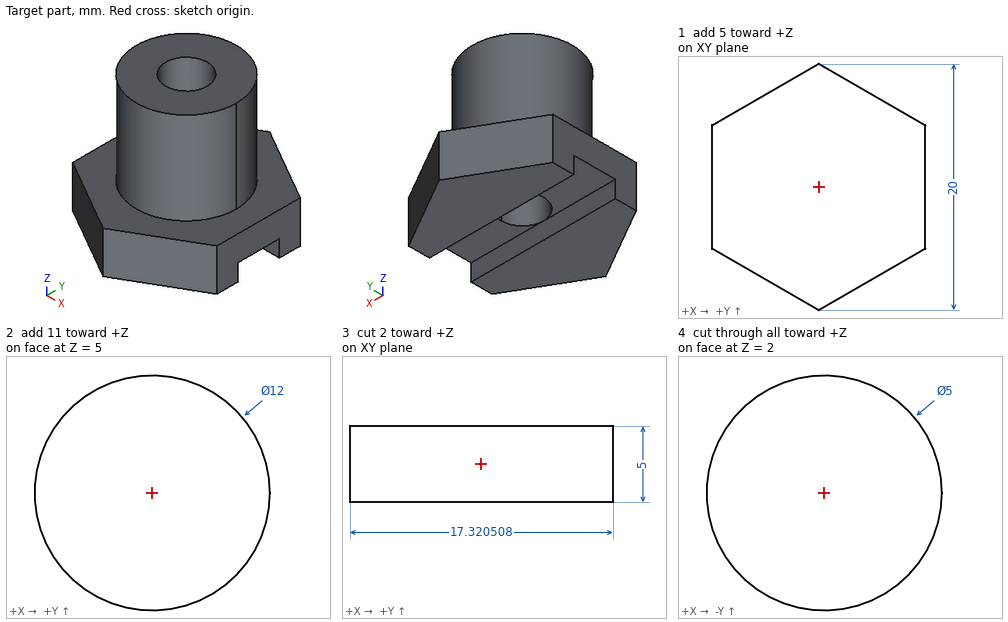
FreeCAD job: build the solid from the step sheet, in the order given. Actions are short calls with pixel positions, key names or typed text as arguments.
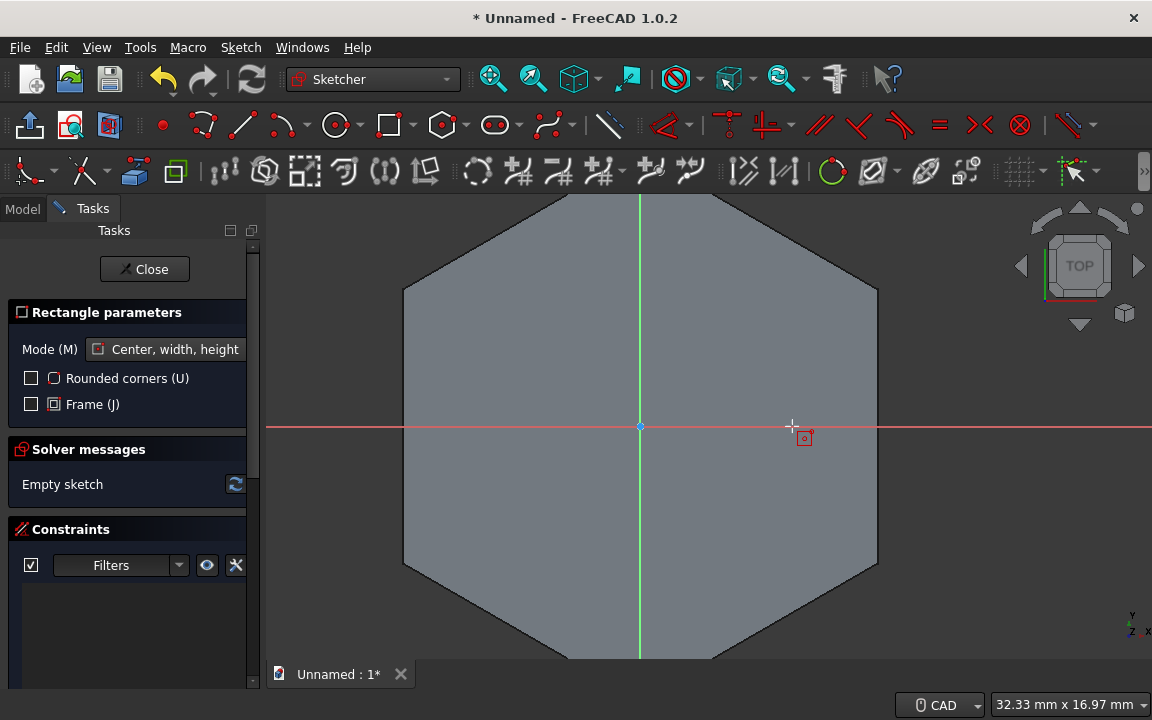
click(640, 426)
click(878, 358)
key(Escape)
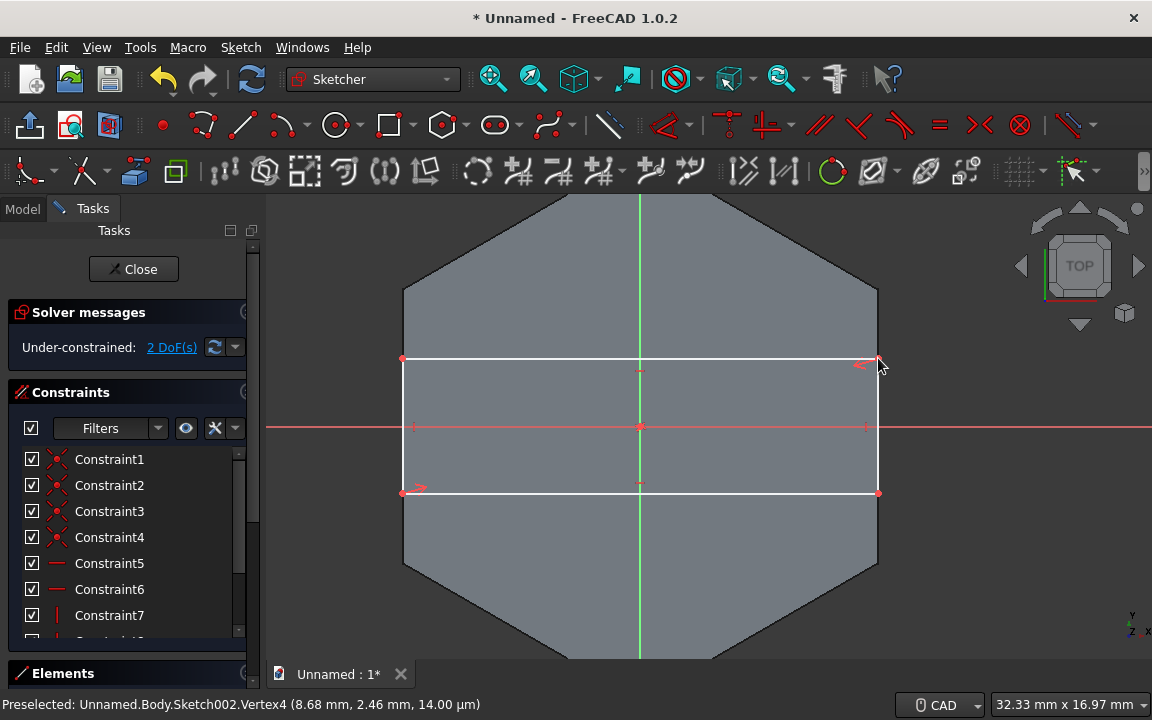
key(d)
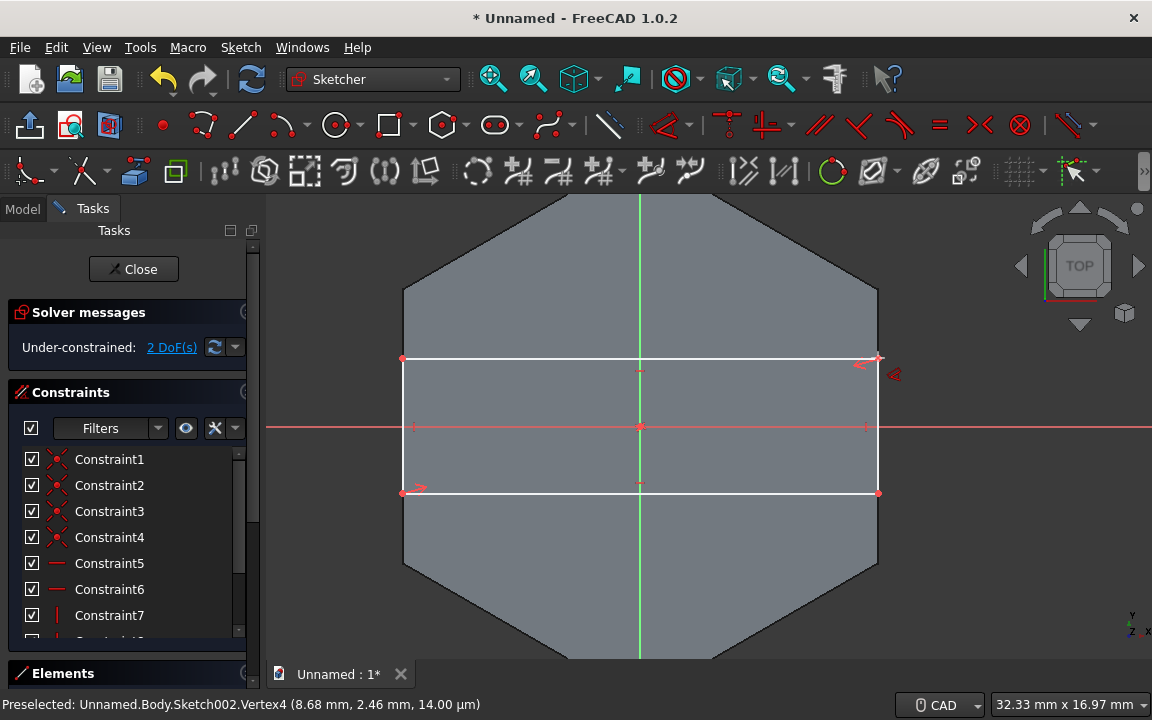
click(878, 453)
click(912, 395)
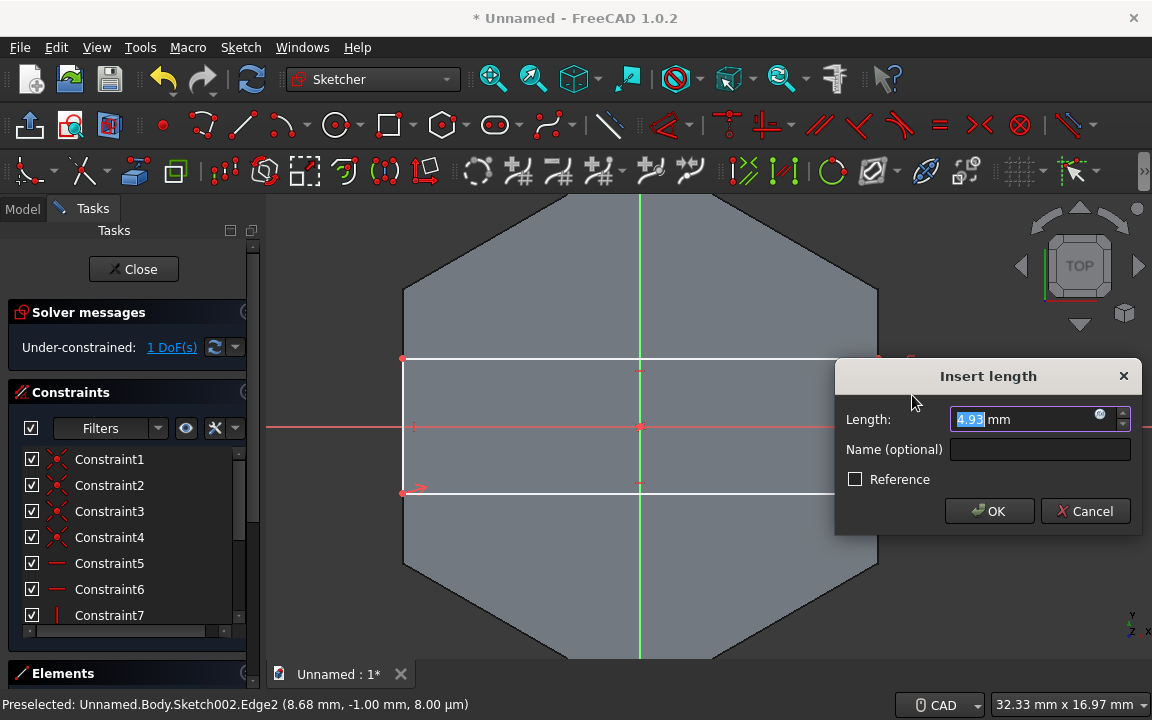
text(5)
key(Return)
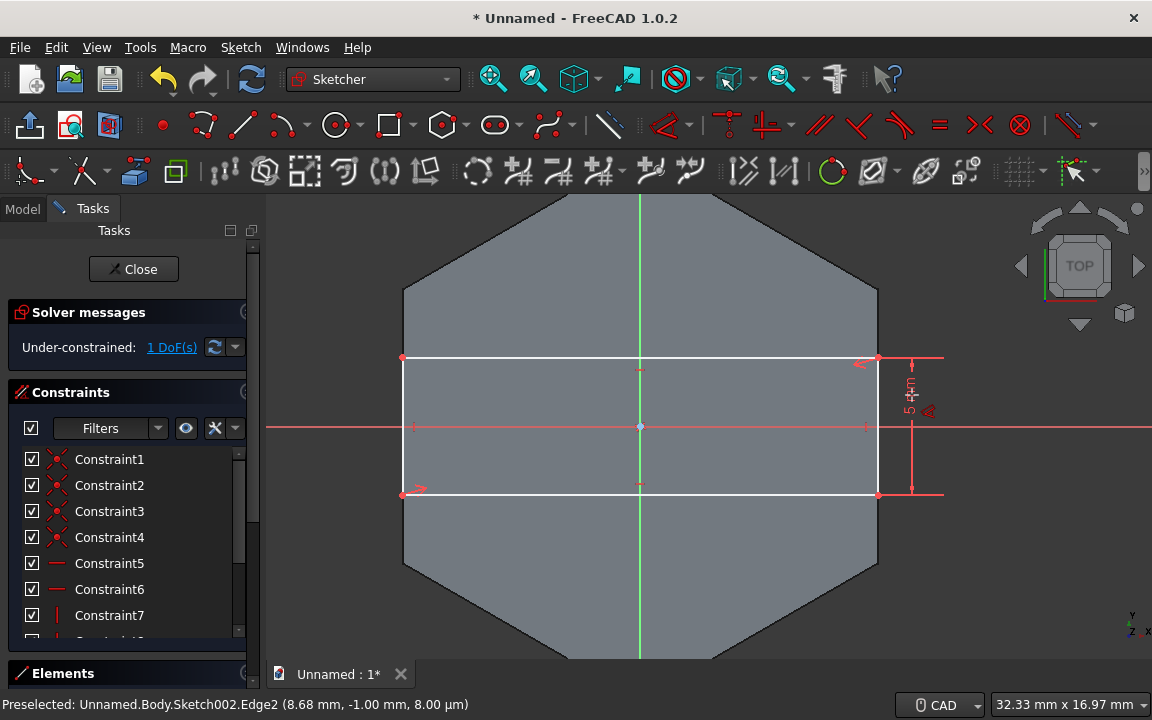
click(545, 495)
click(531, 529)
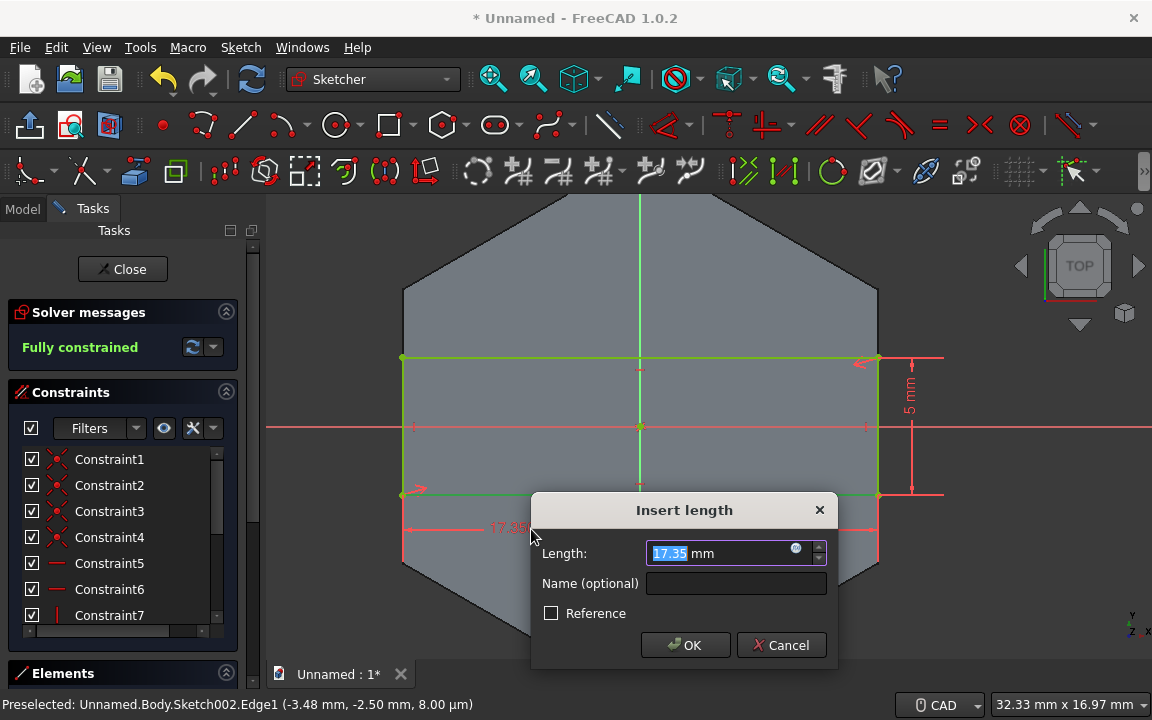
text(17.320508)
key(Return)
key(Escape)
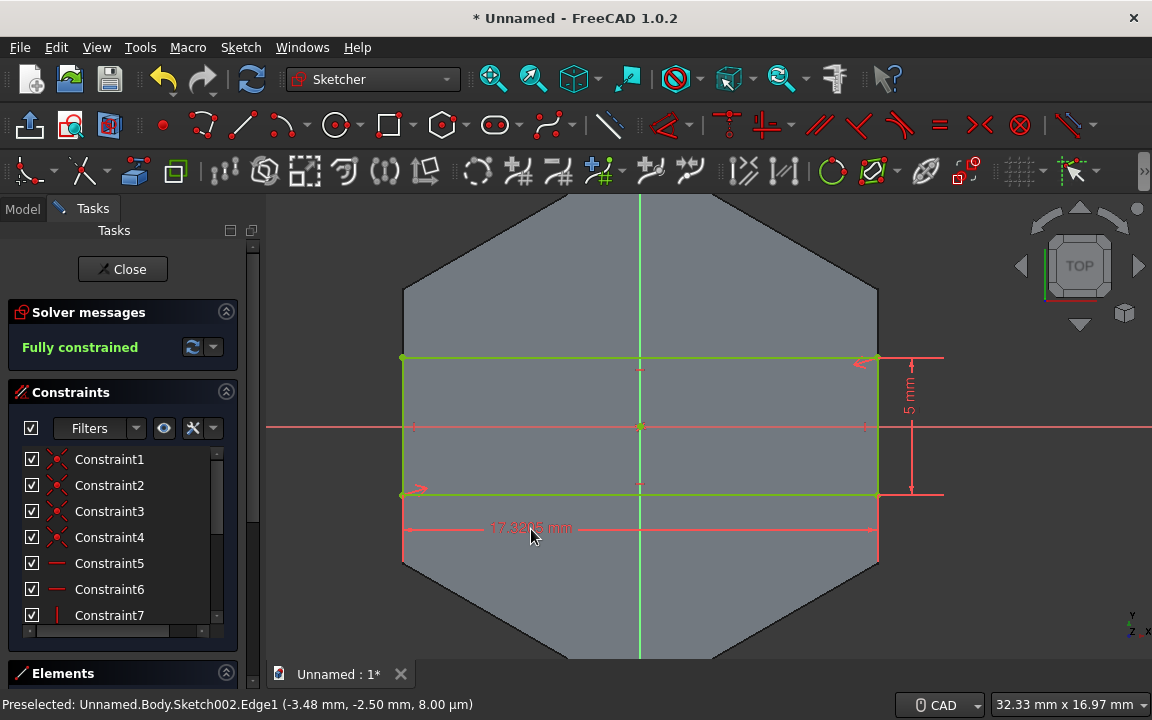
click(123, 269)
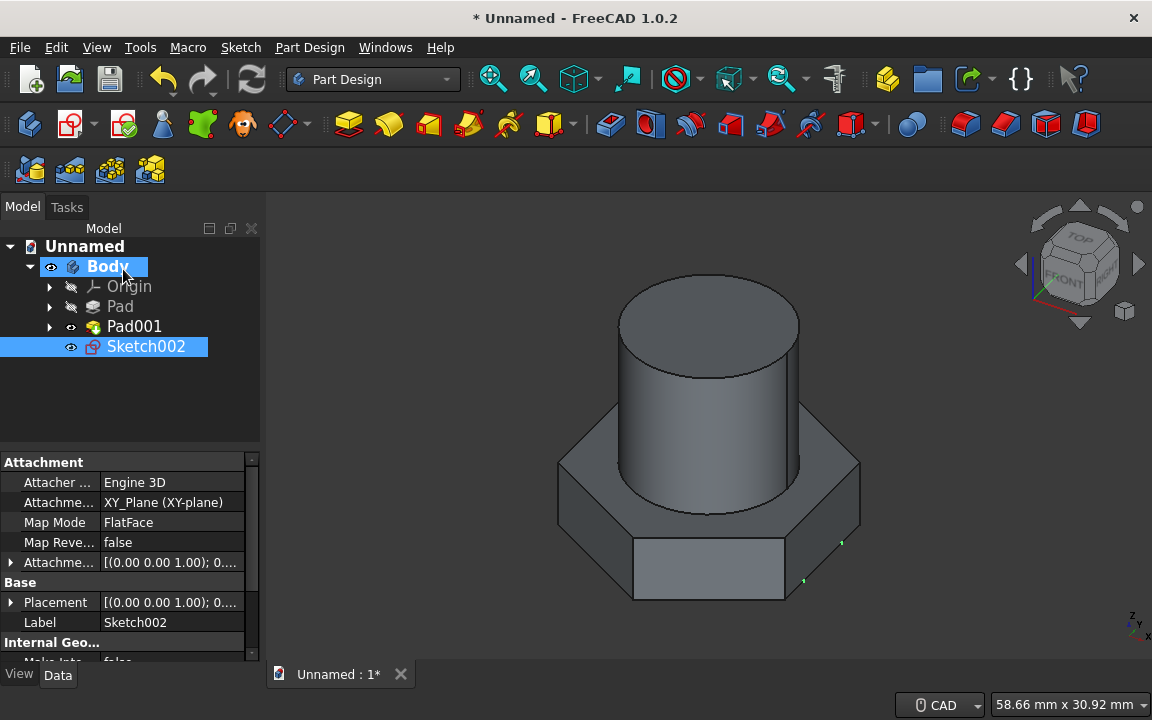
click(612, 124)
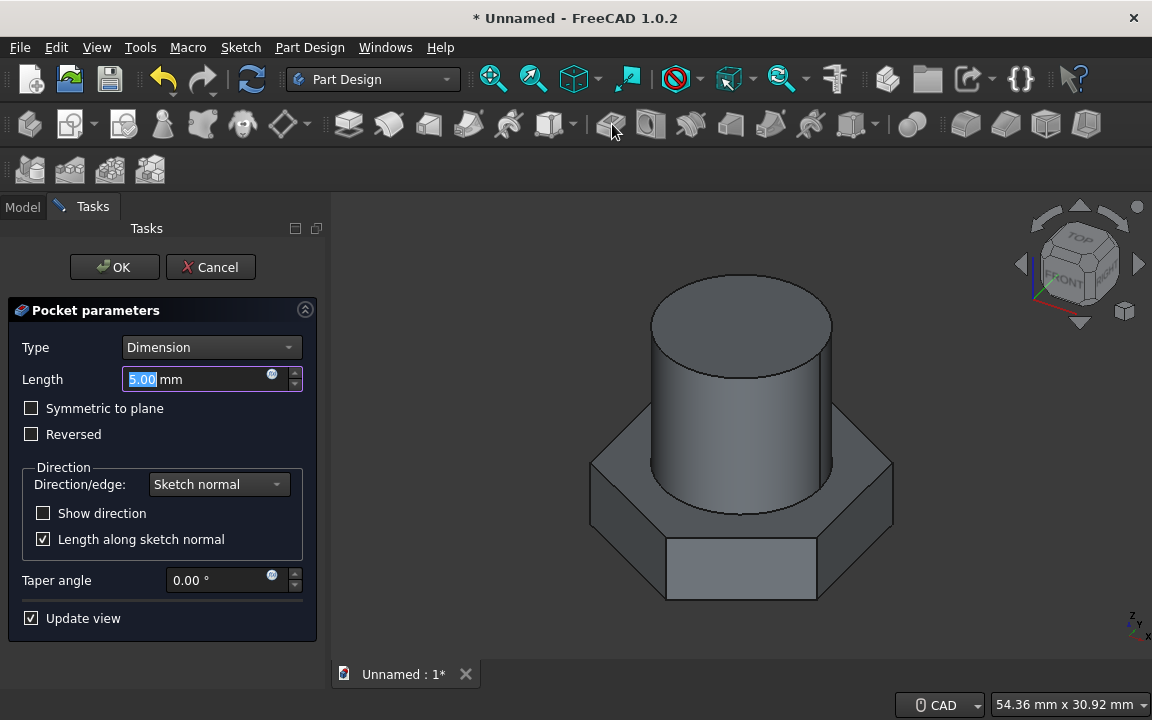
text(2)
key(Tab)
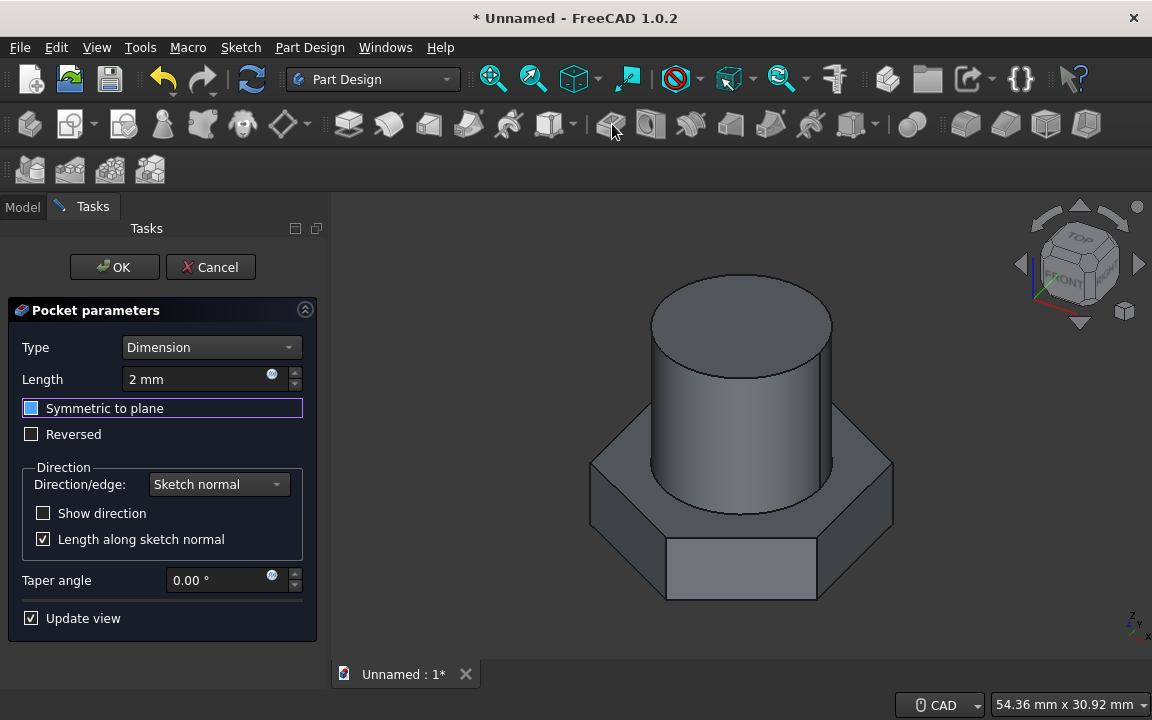
click(30, 434)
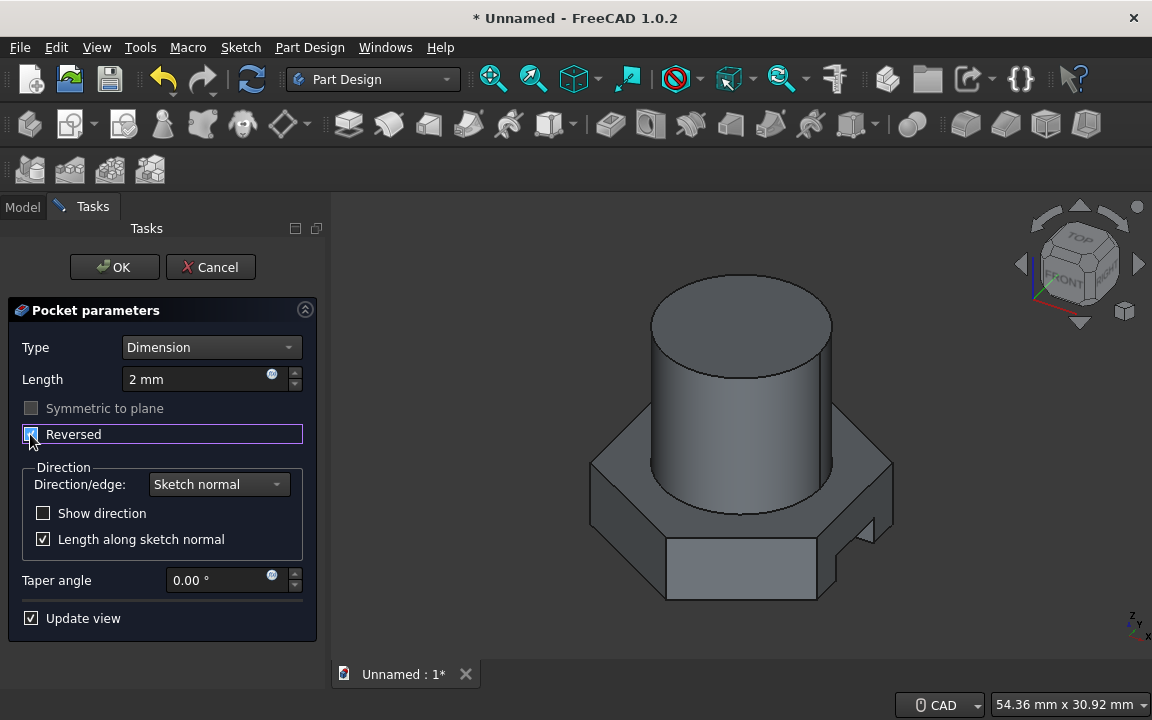
click(115, 267)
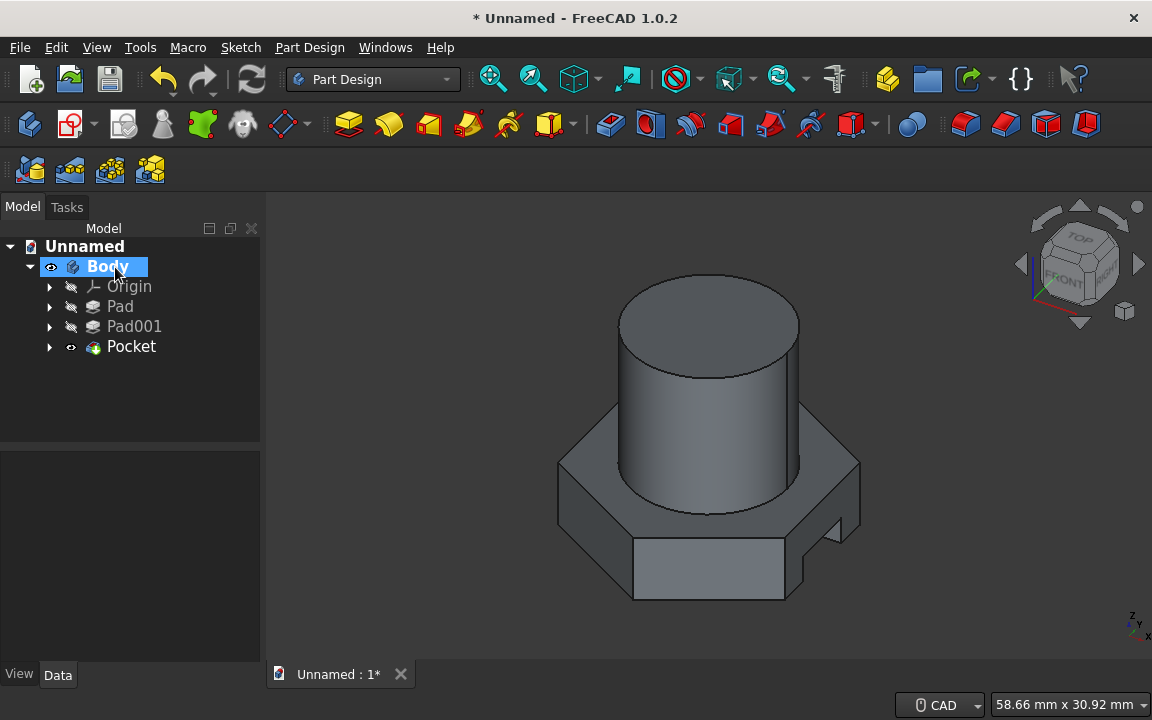
key(5)